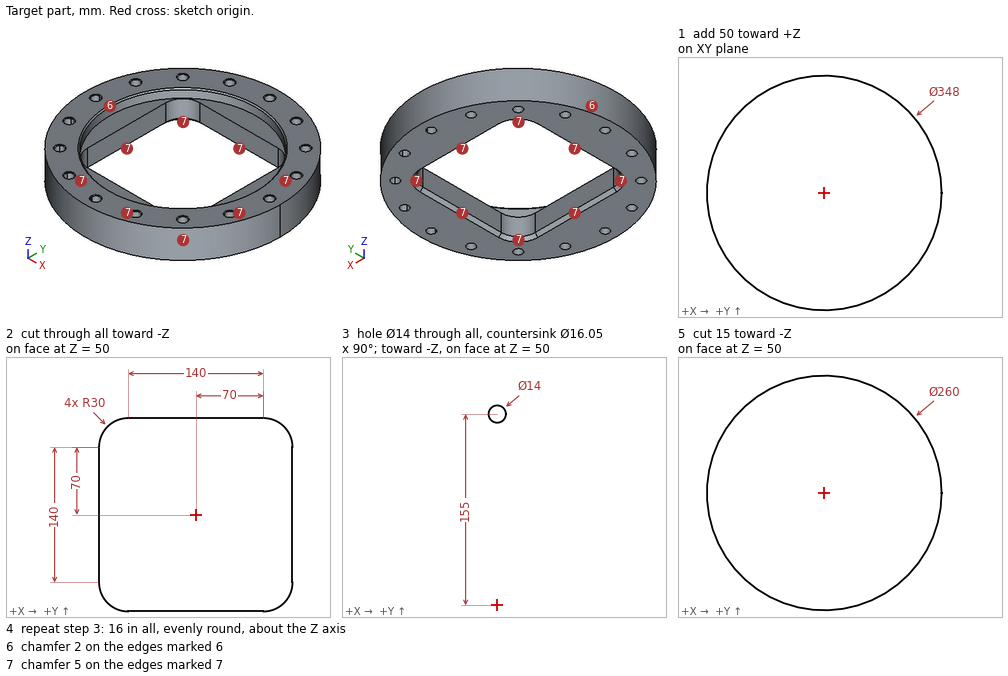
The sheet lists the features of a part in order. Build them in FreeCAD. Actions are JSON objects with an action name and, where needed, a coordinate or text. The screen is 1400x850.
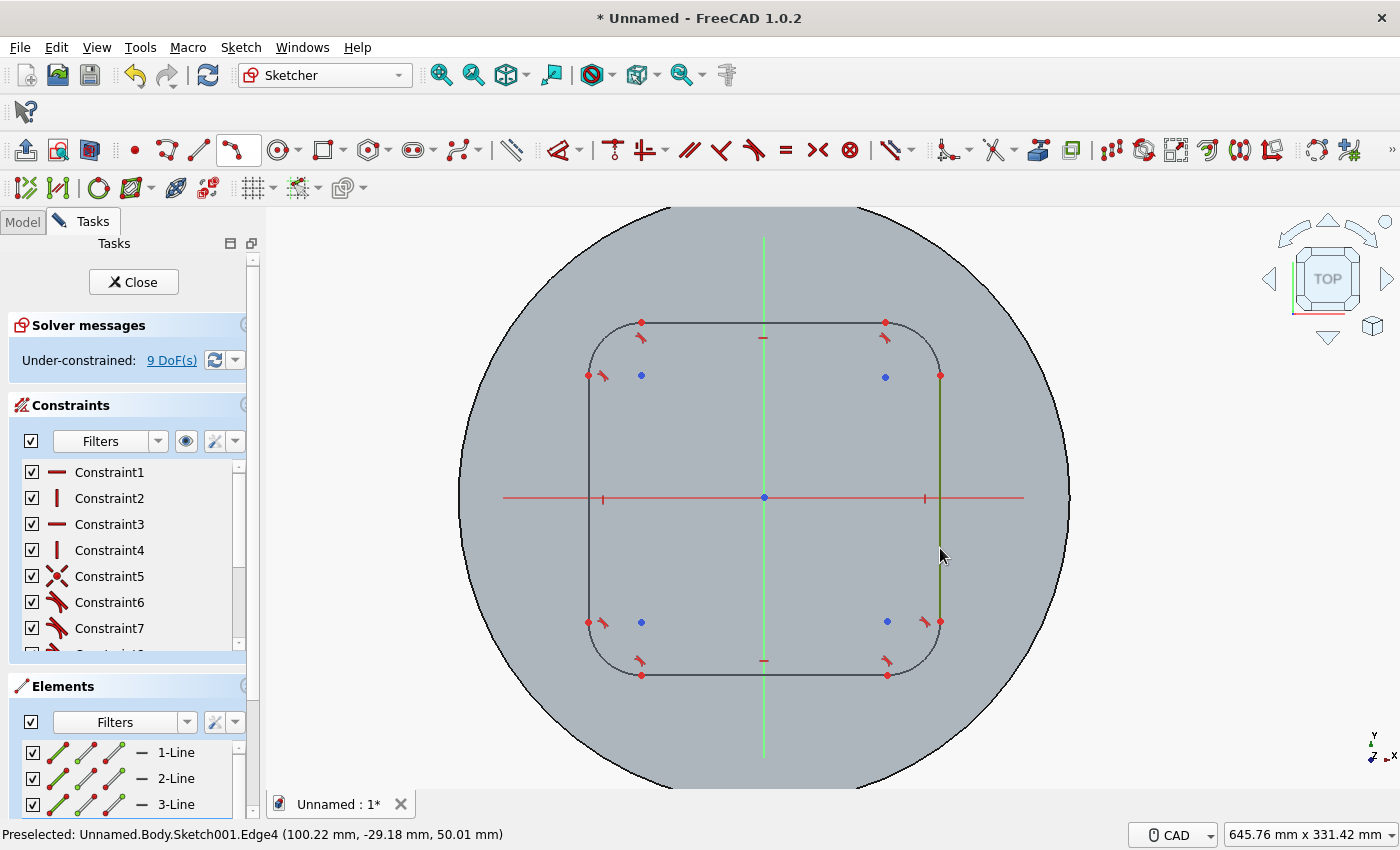
{"action": "left_click", "coordinate": [934, 352]}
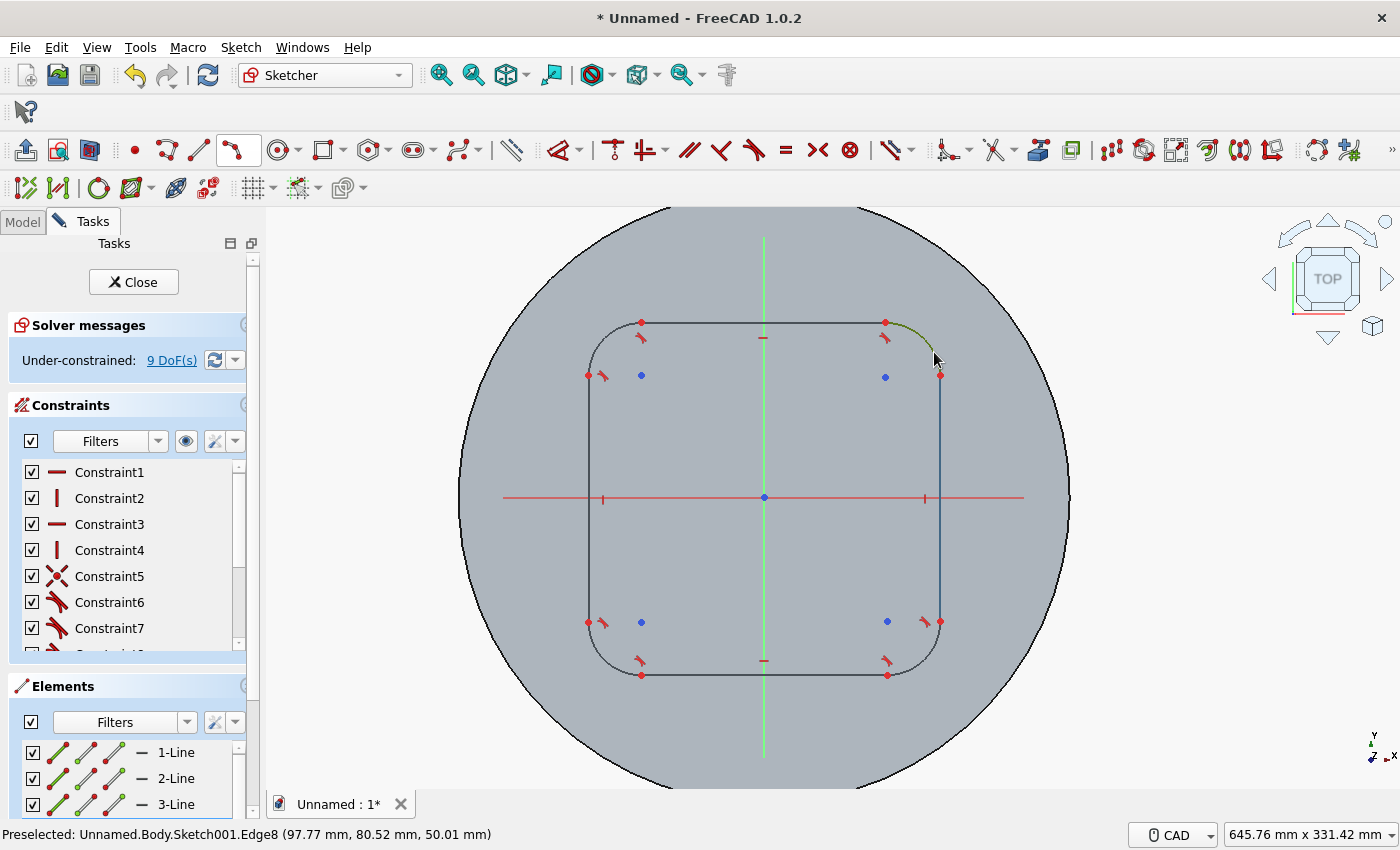
{"action": "left_click", "coordinate": [754, 150]}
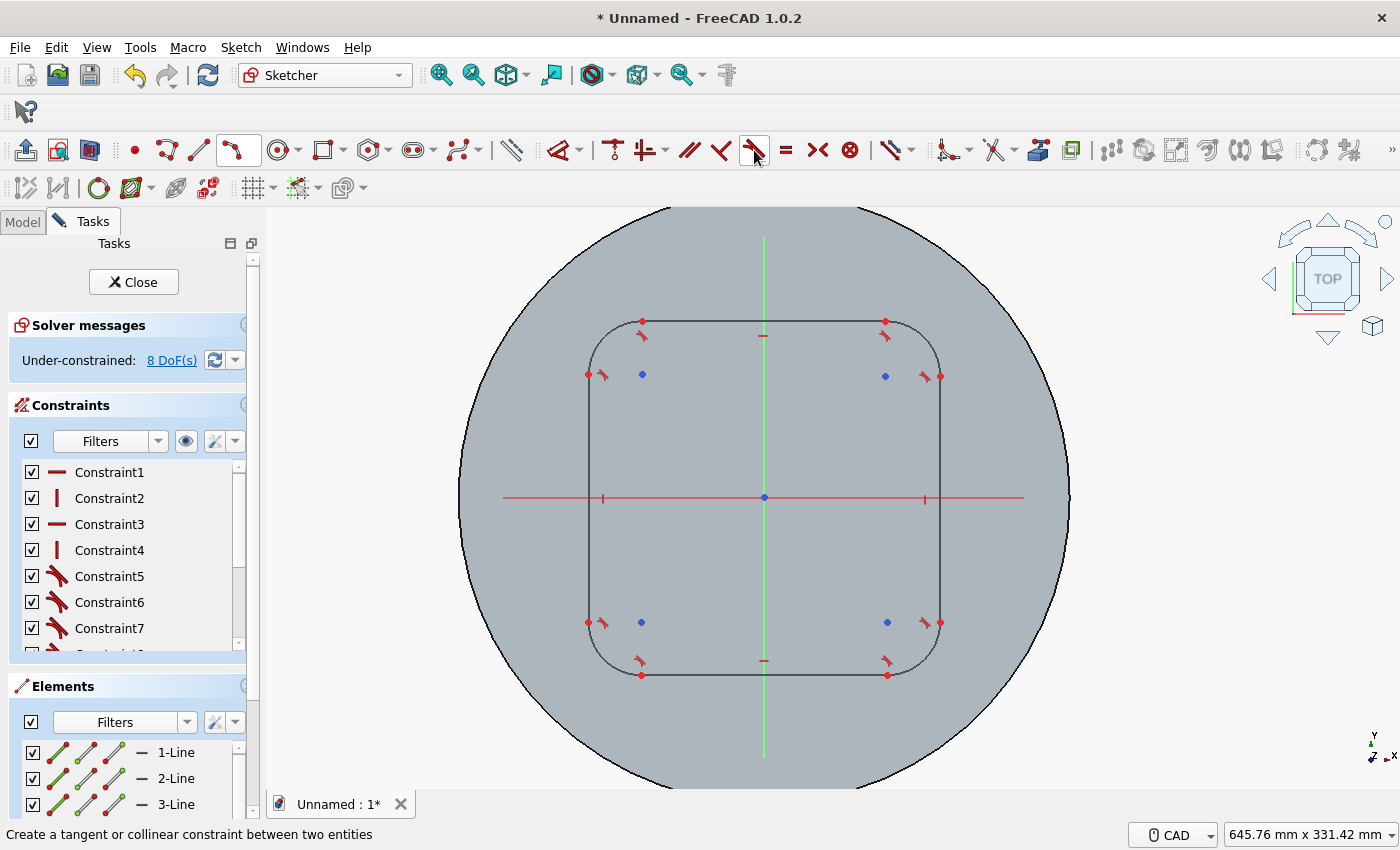
{"action": "left_click", "coordinate": [618, 327]}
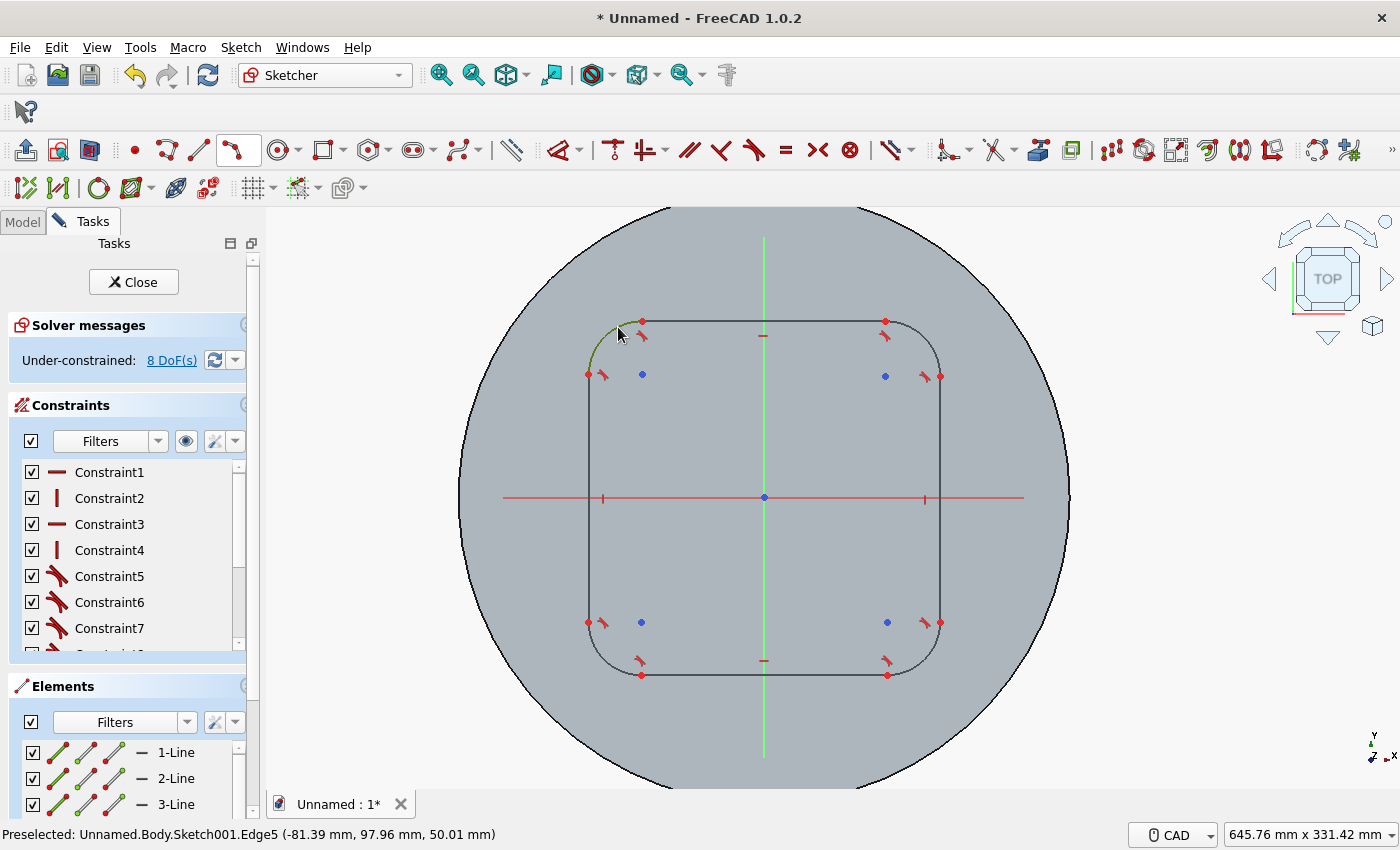
{"action": "left_click", "coordinate": [595, 647]}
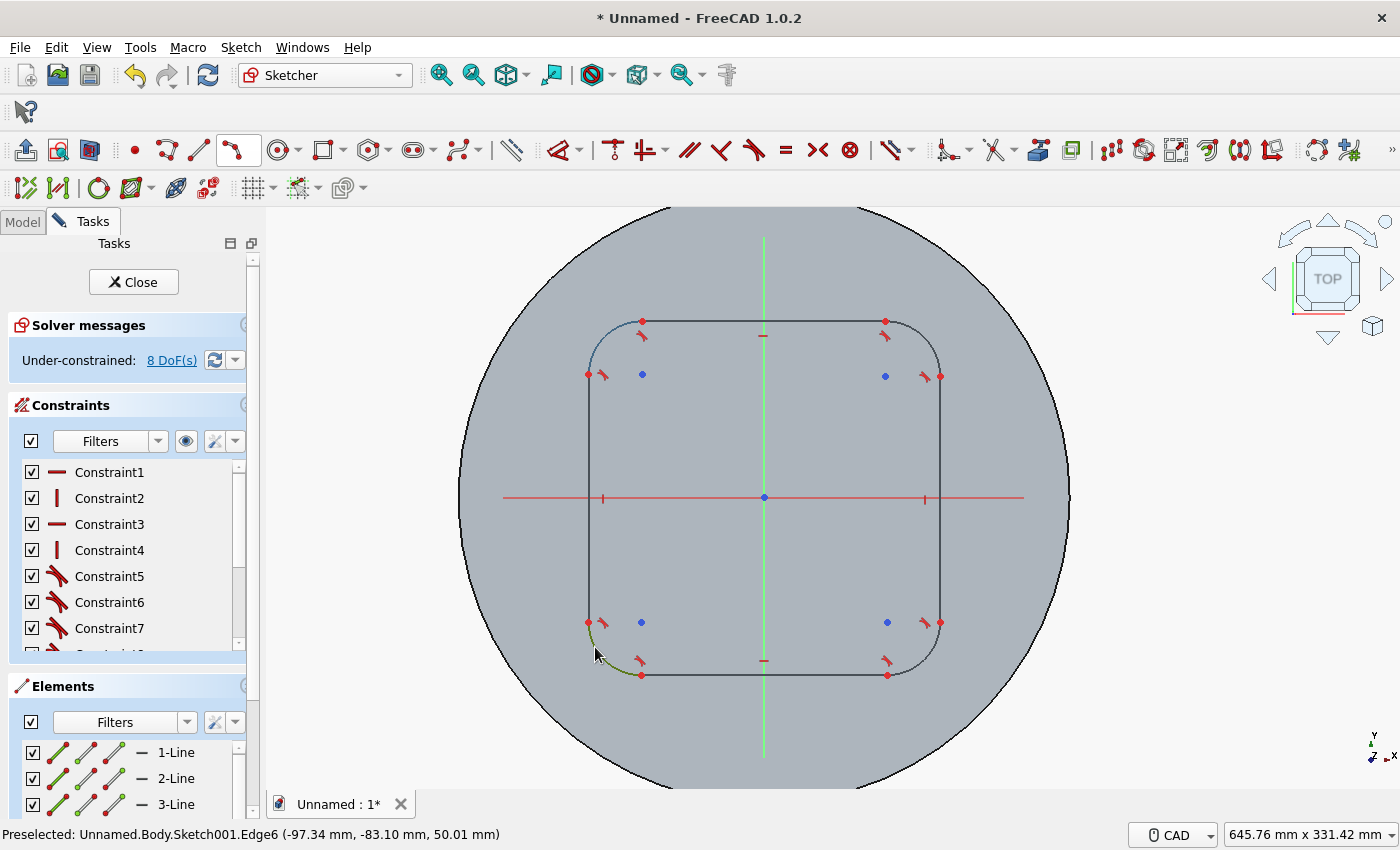
{"action": "left_click", "coordinate": [911, 669]}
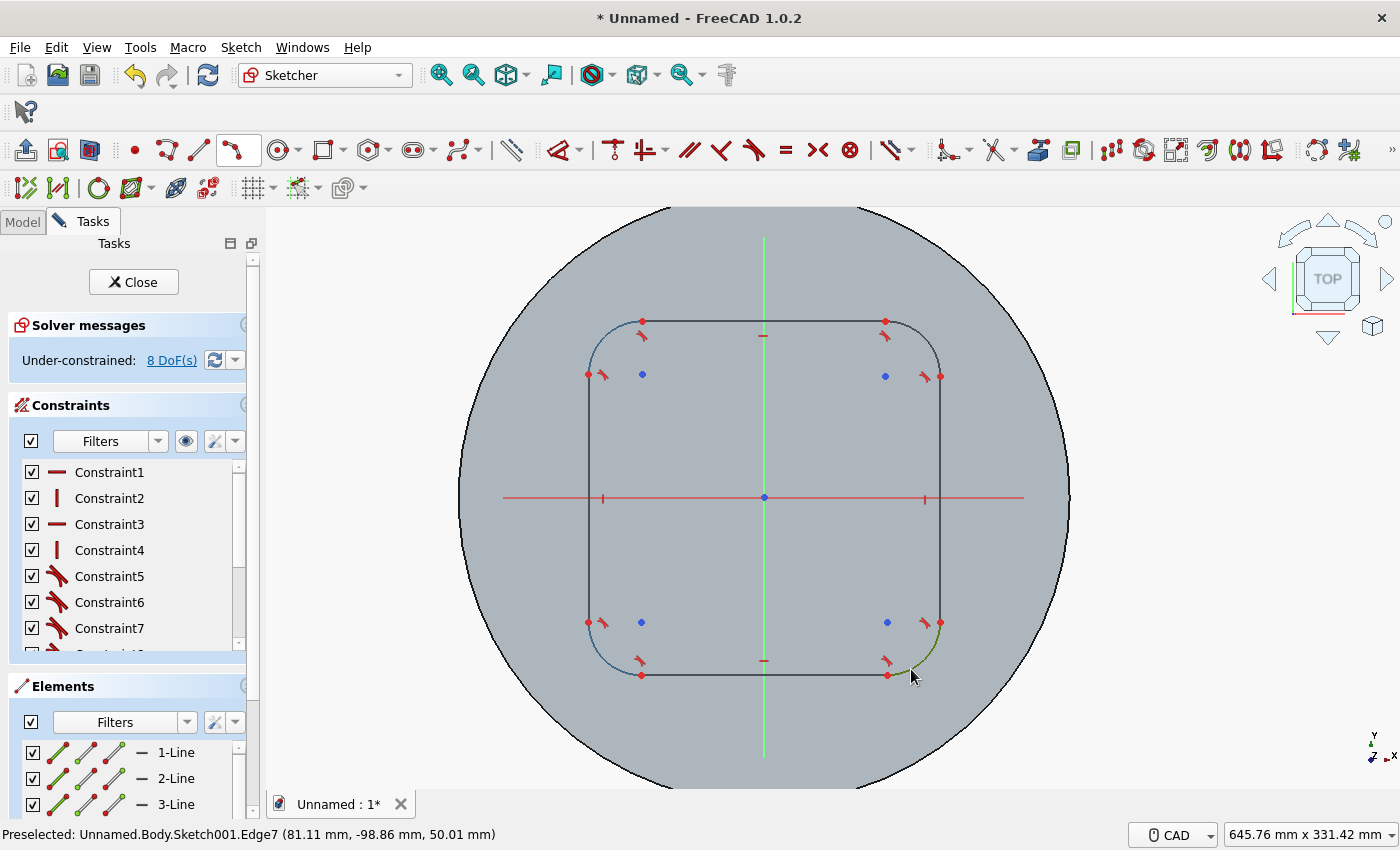
{"action": "left_click", "coordinate": [934, 351]}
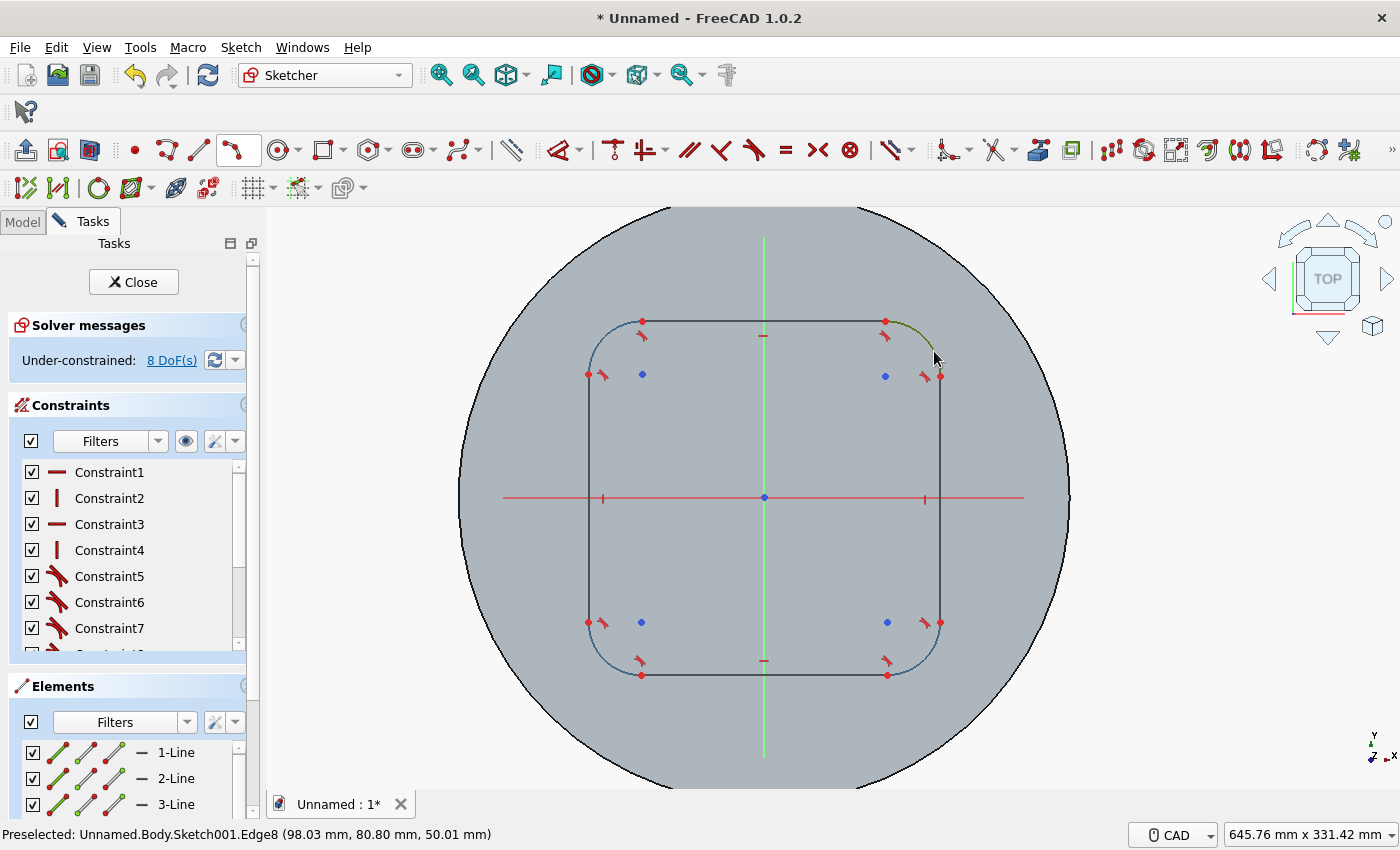
{"action": "left_click", "coordinate": [786, 150]}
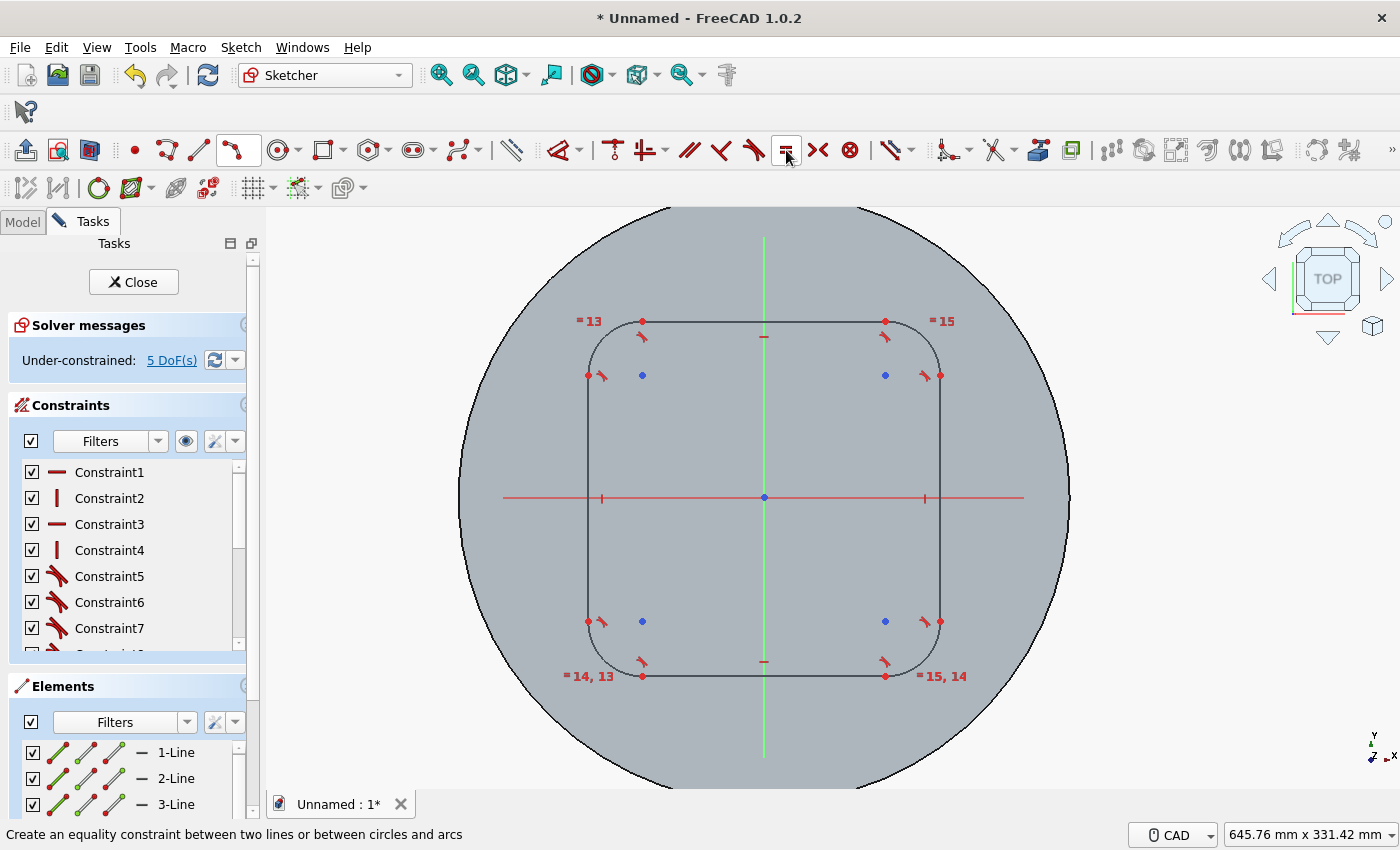
{"action": "left_click", "coordinate": [558, 150]}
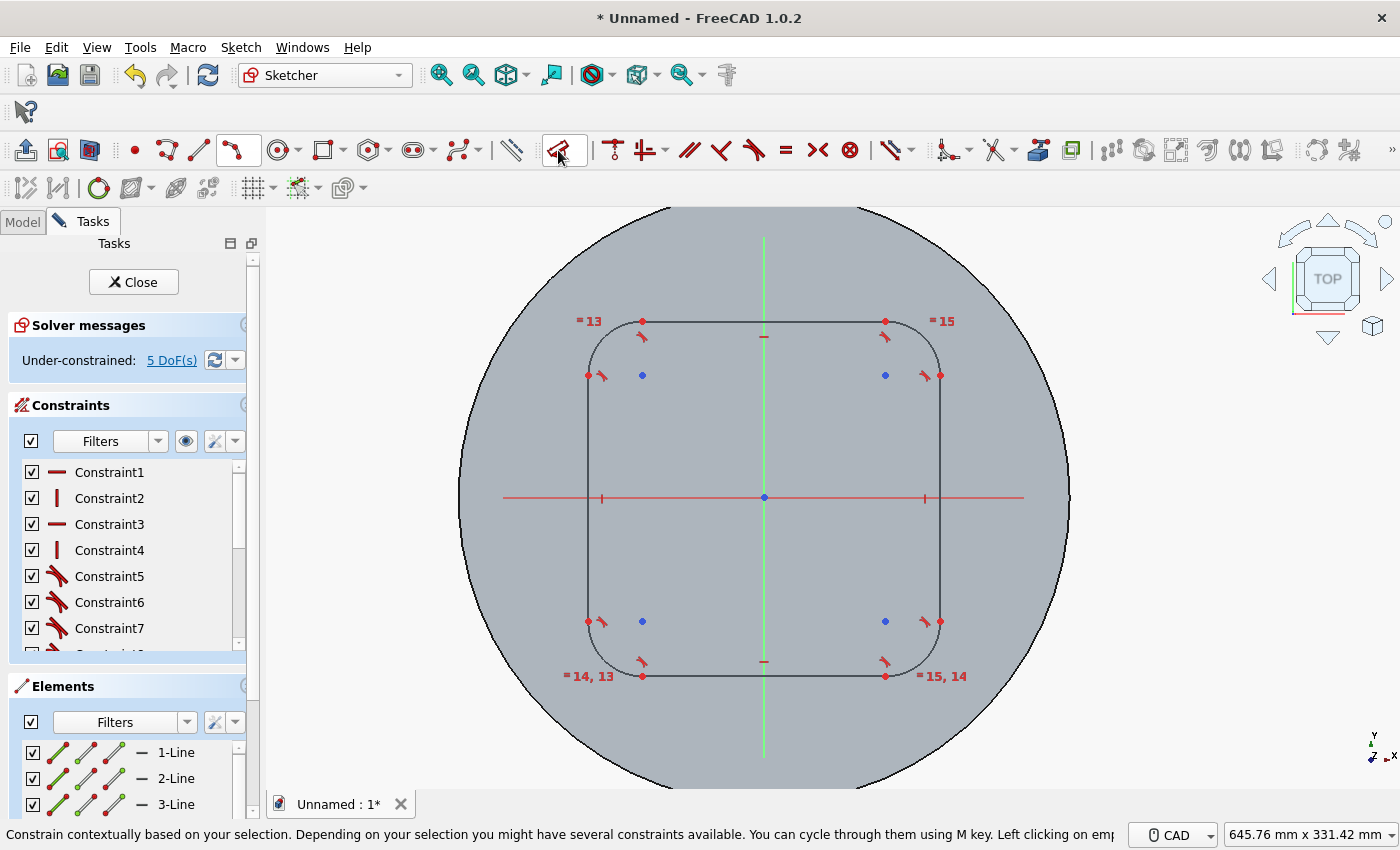
{"action": "left_click", "coordinate": [618, 328]}
{"action": "left_click", "coordinate": [603, 300]}